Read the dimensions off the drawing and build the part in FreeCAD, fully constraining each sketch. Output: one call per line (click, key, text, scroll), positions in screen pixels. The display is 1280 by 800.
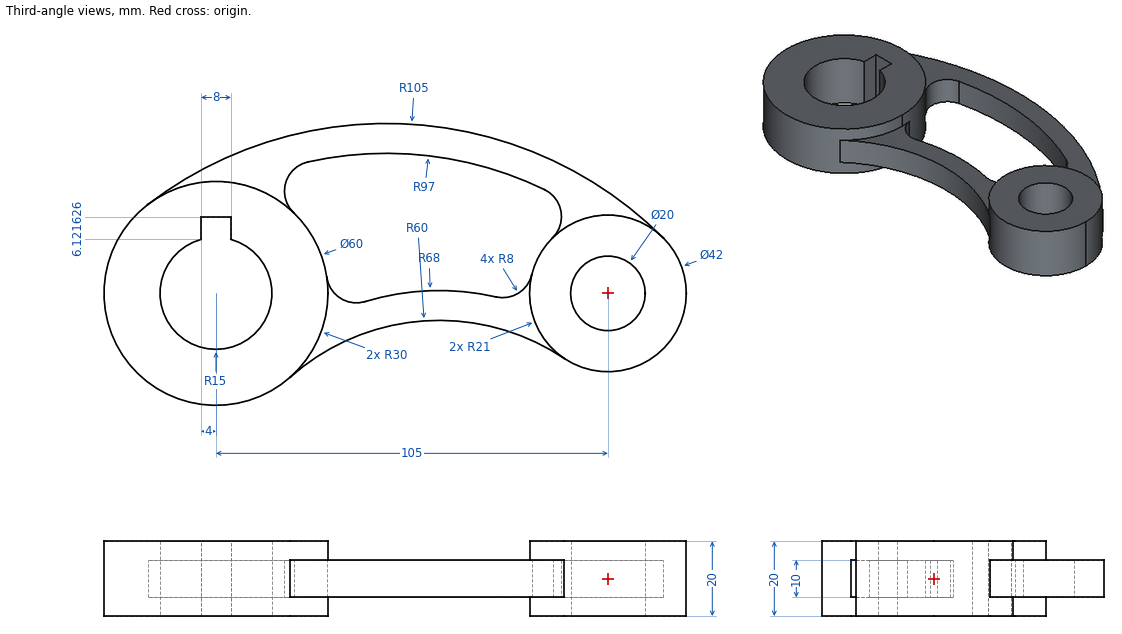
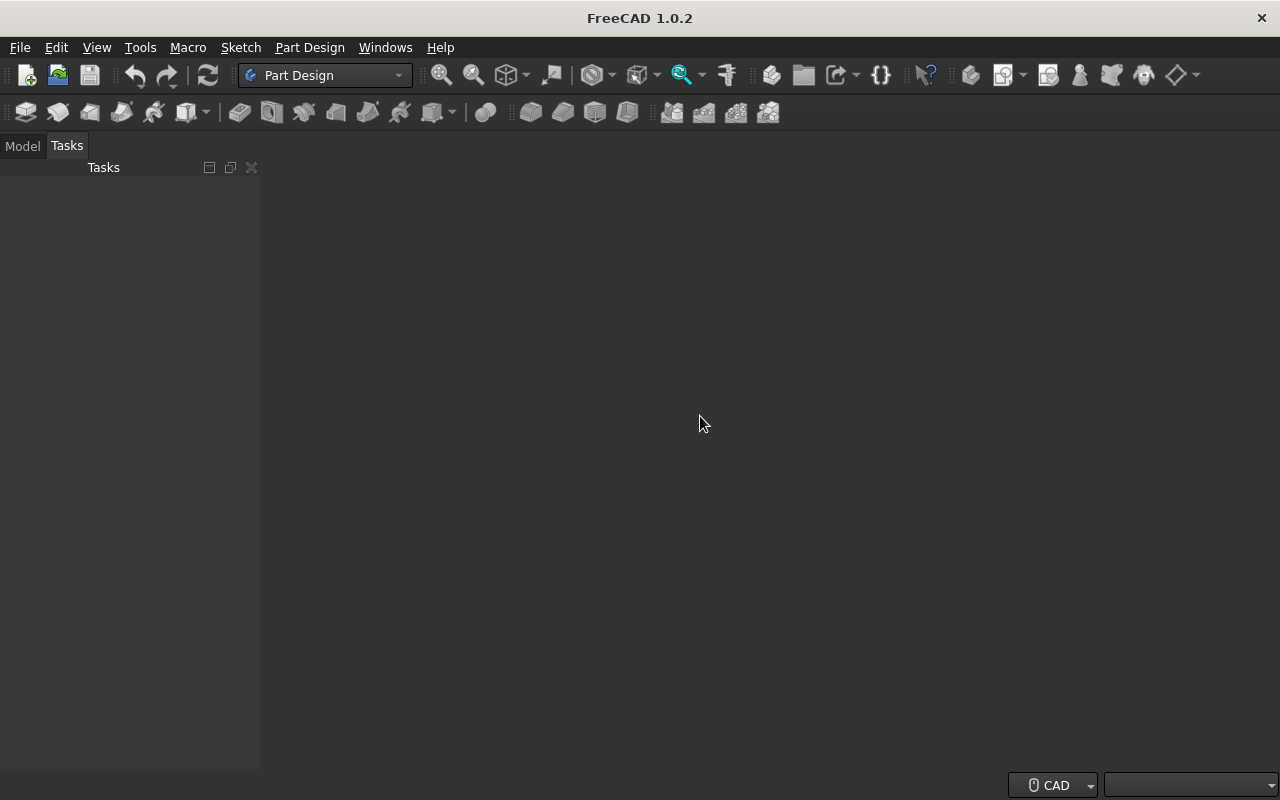
click(26, 76)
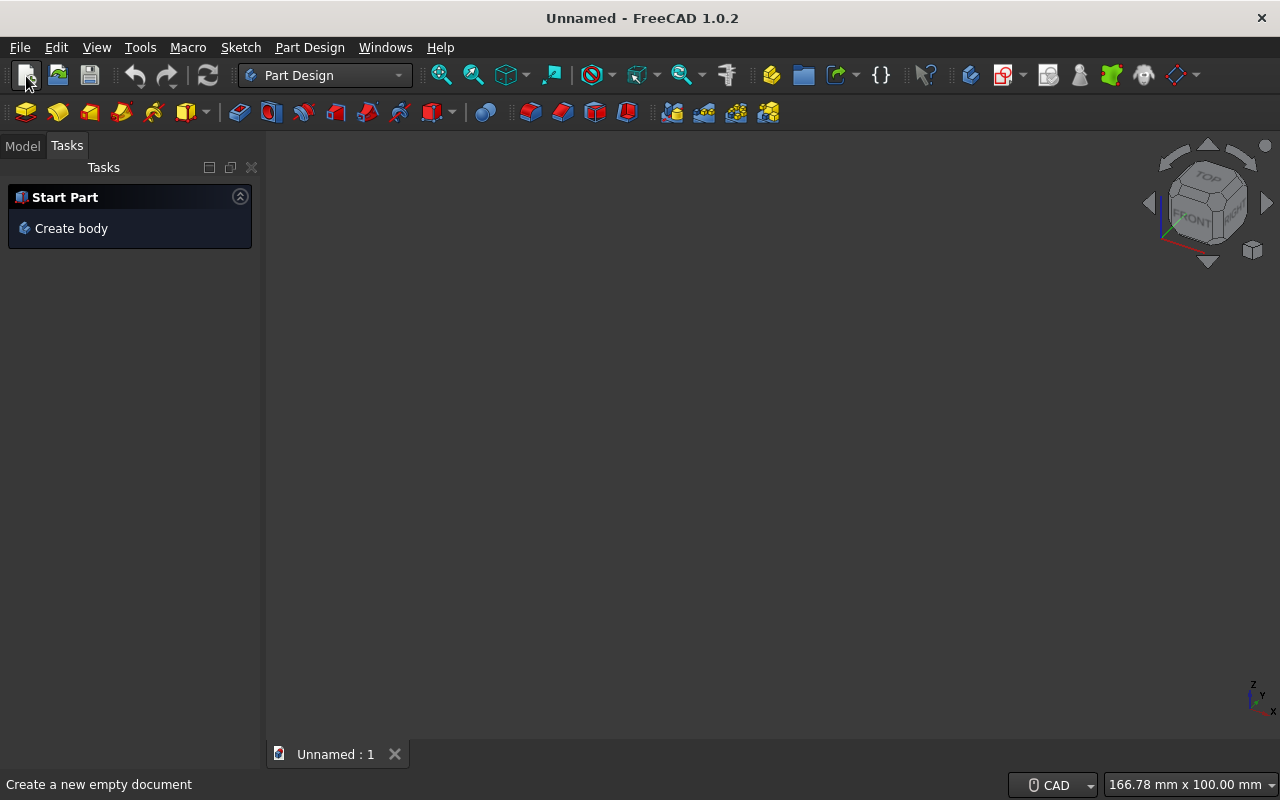
click(1004, 76)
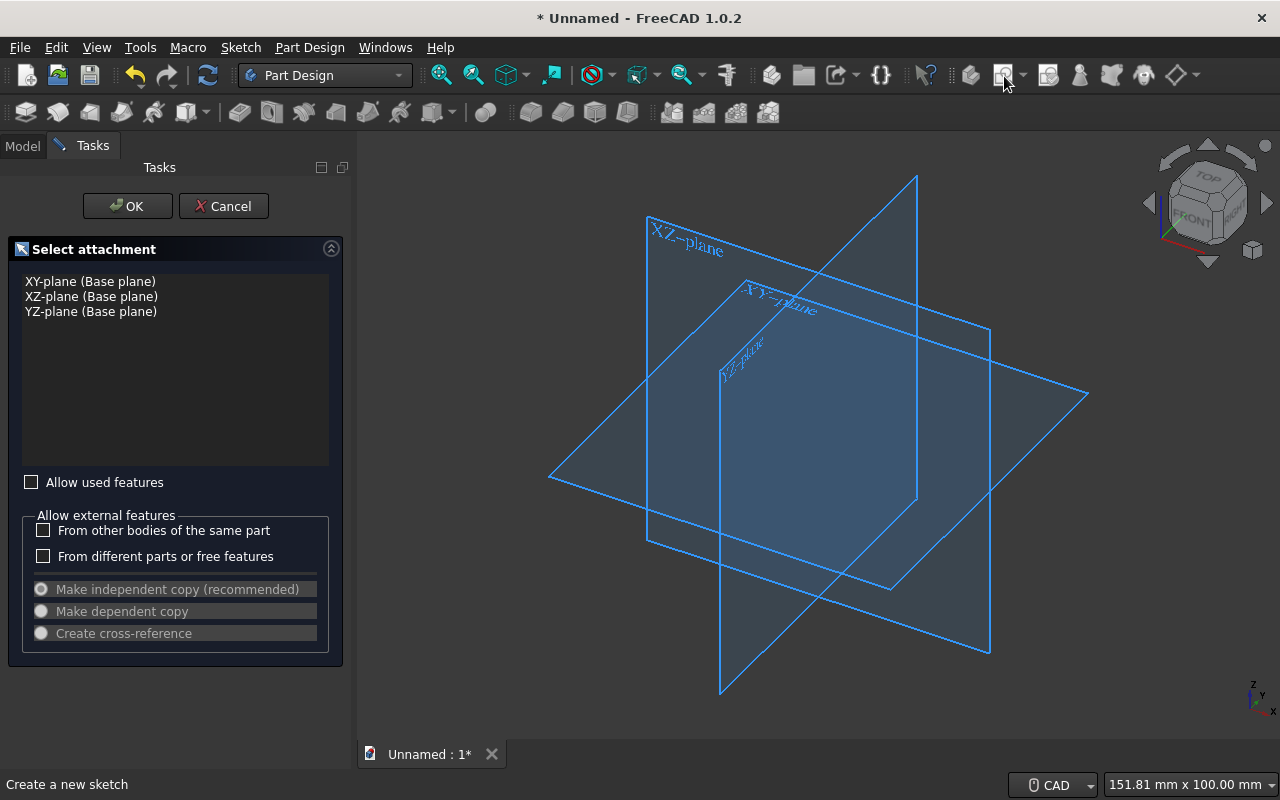
click(82, 282)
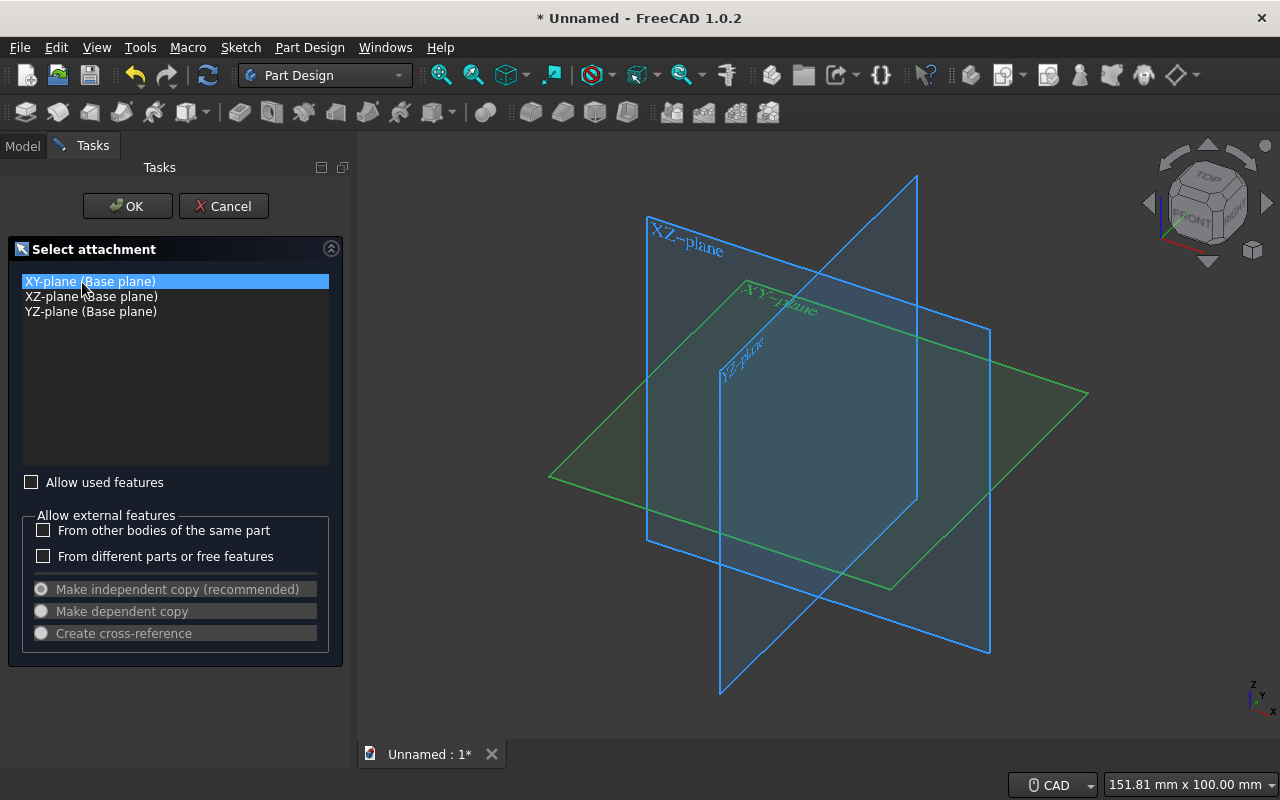
click(128, 206)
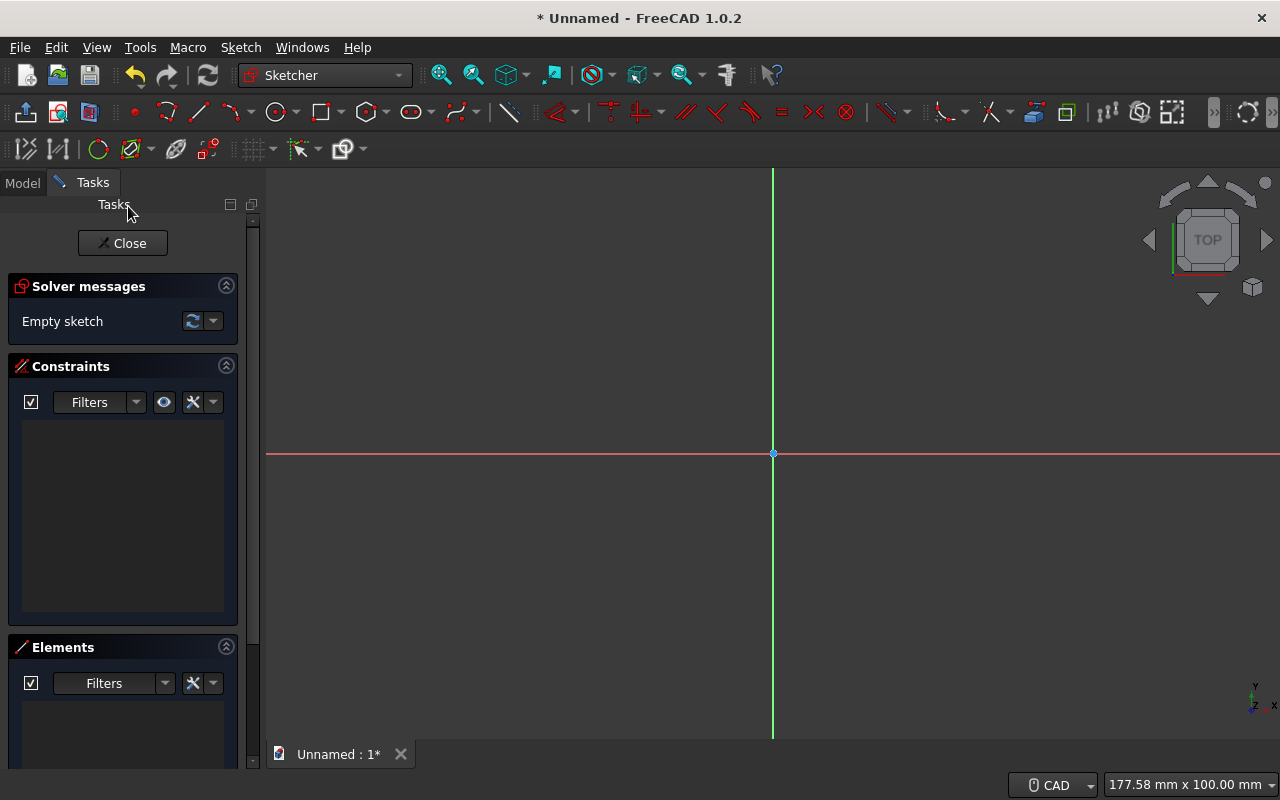
scroll(1115, 453, down, 2)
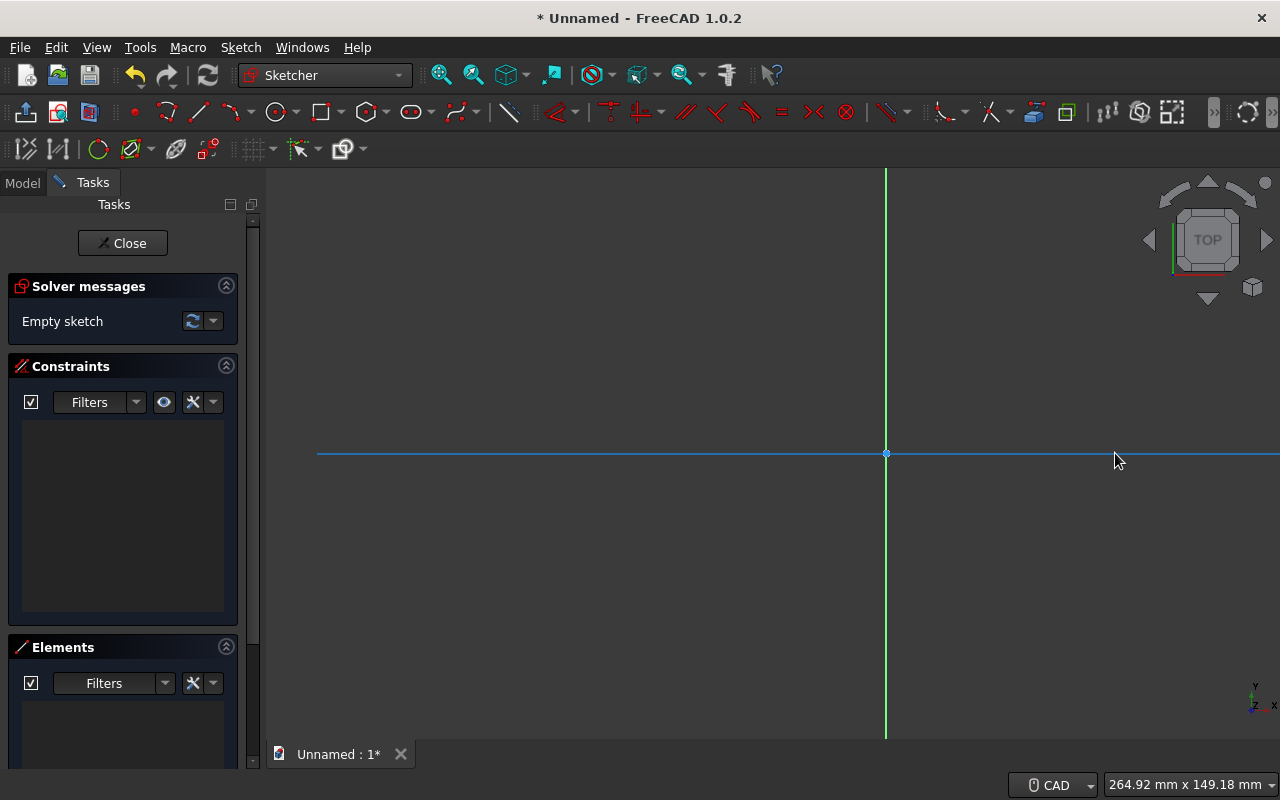
key(g)
key(m)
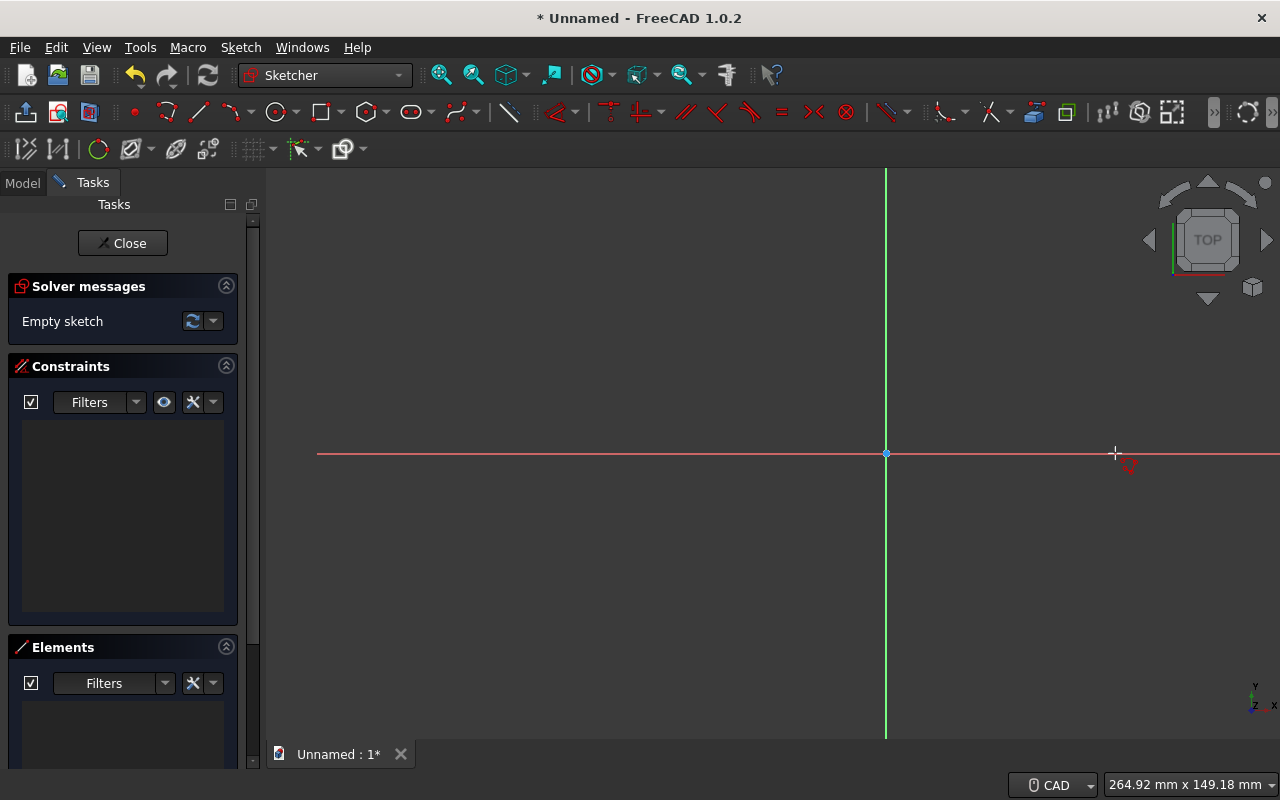
click(469, 398)
click(469, 375)
click(499, 375)
click(499, 398)
right_click(499, 398)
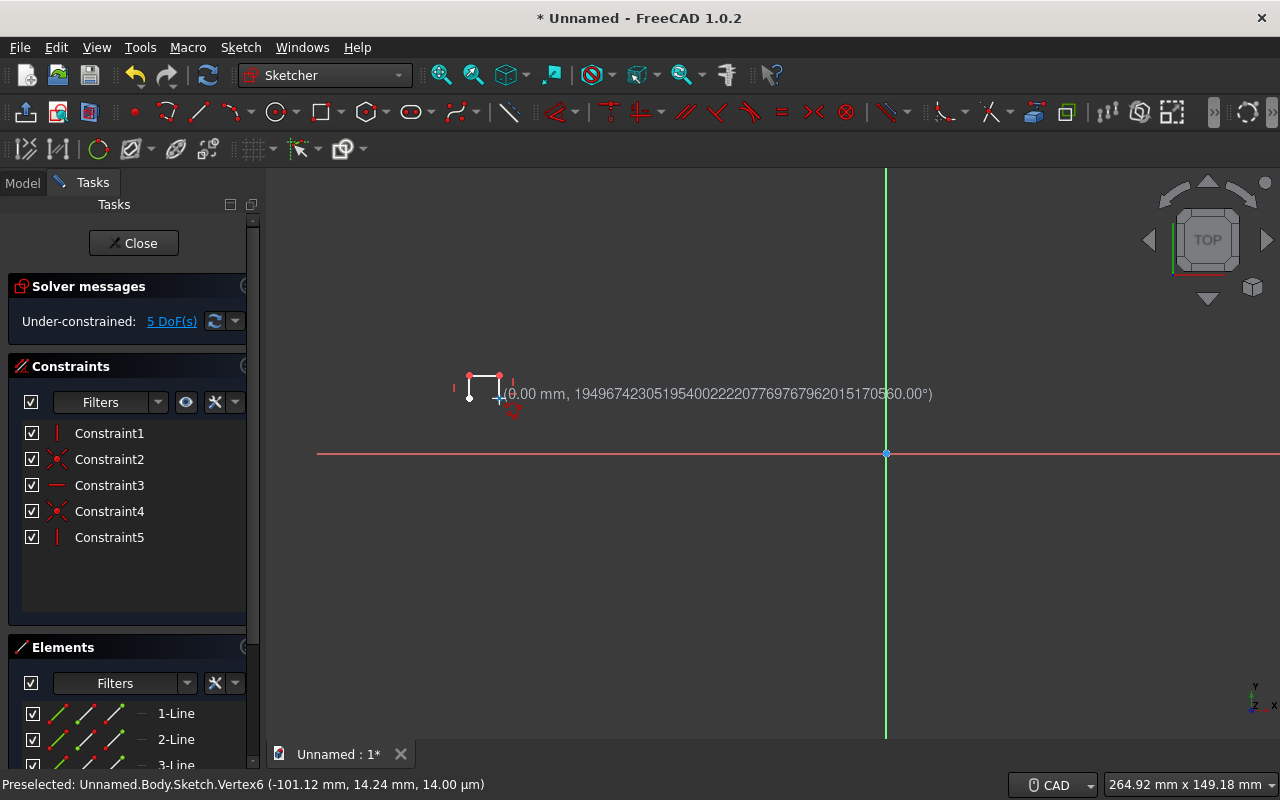
key(g)
key(3)
key(a)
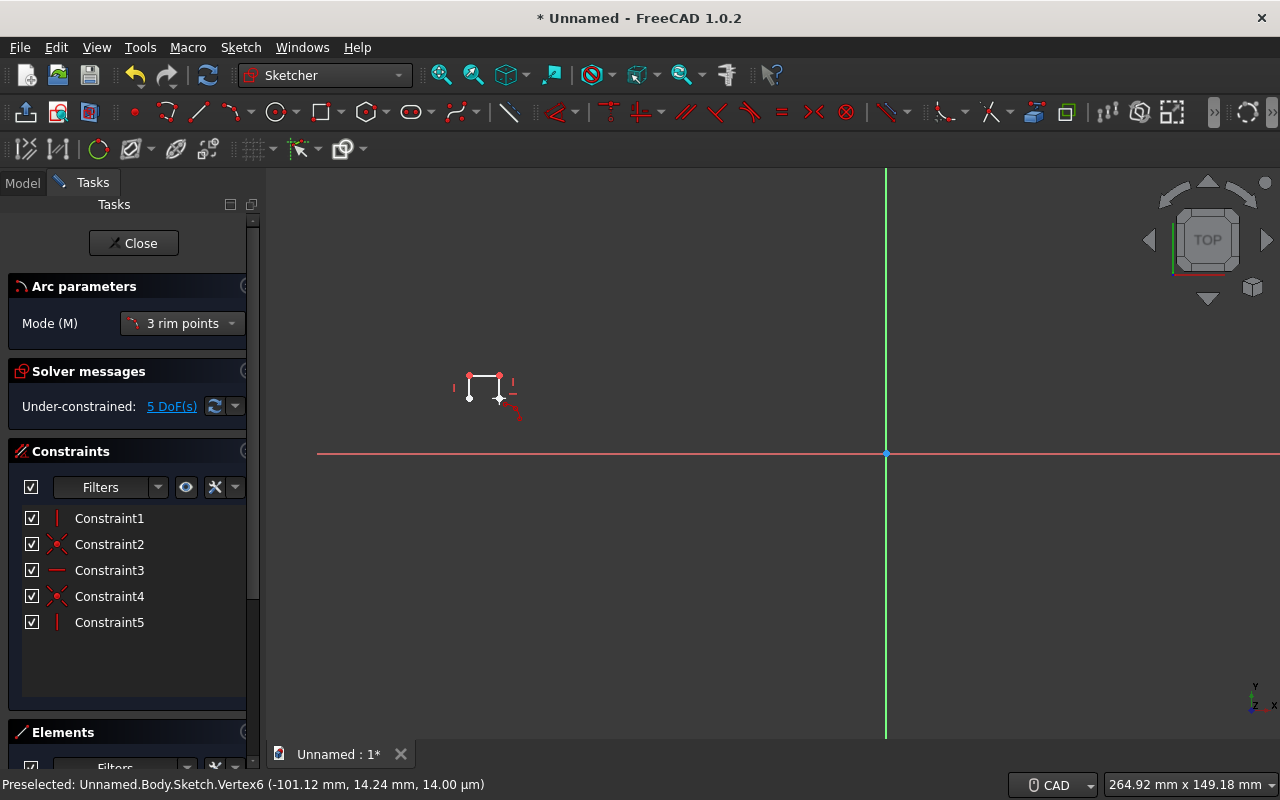
scroll(499, 398, up, 2)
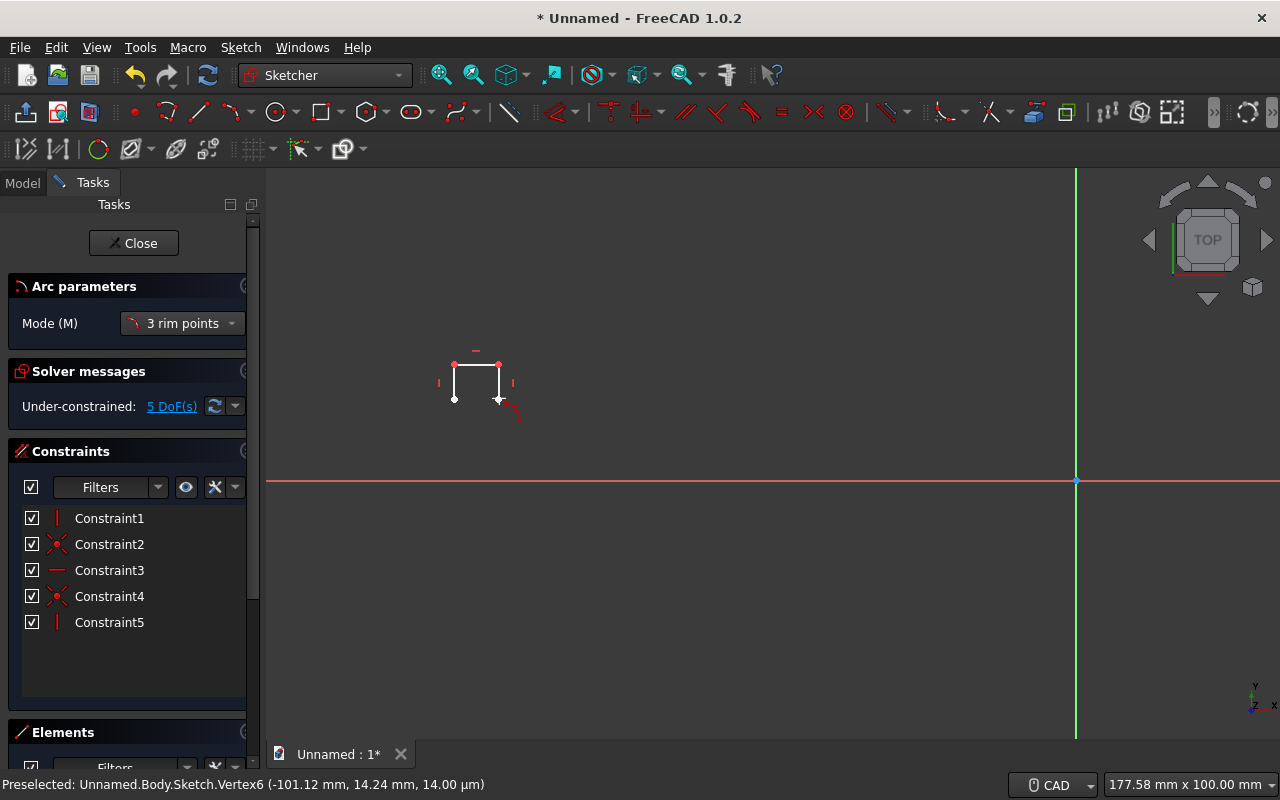
click(499, 399)
click(454, 399)
click(477, 566)